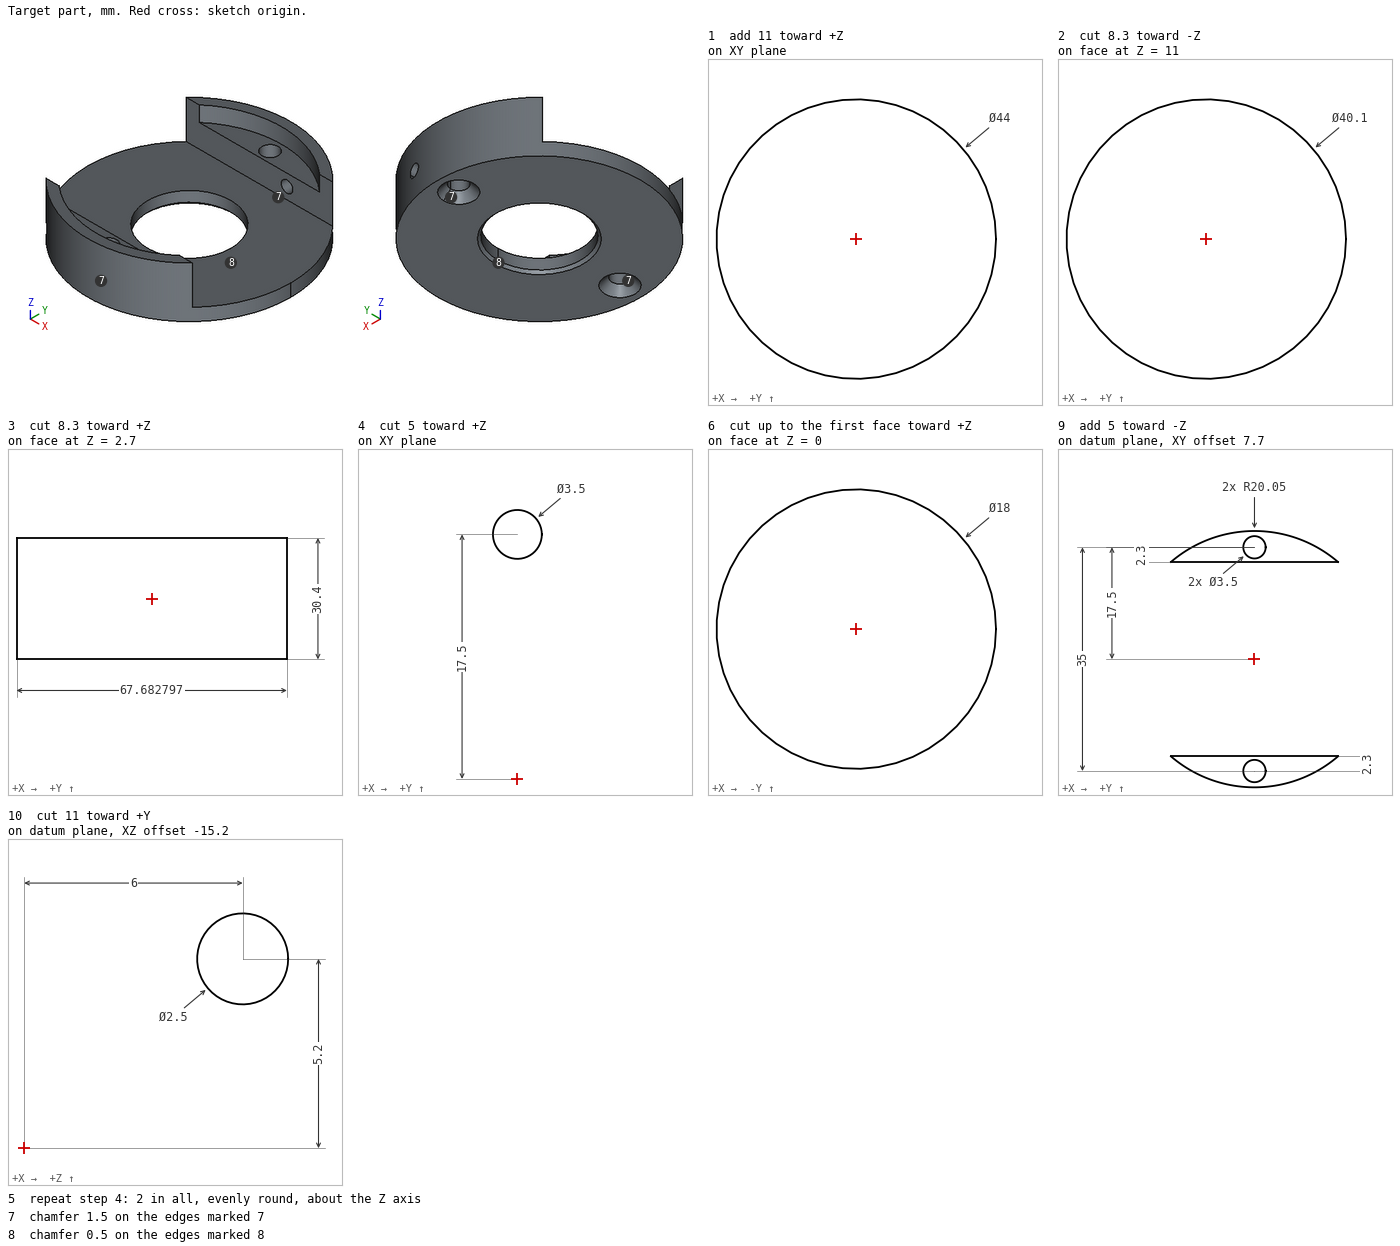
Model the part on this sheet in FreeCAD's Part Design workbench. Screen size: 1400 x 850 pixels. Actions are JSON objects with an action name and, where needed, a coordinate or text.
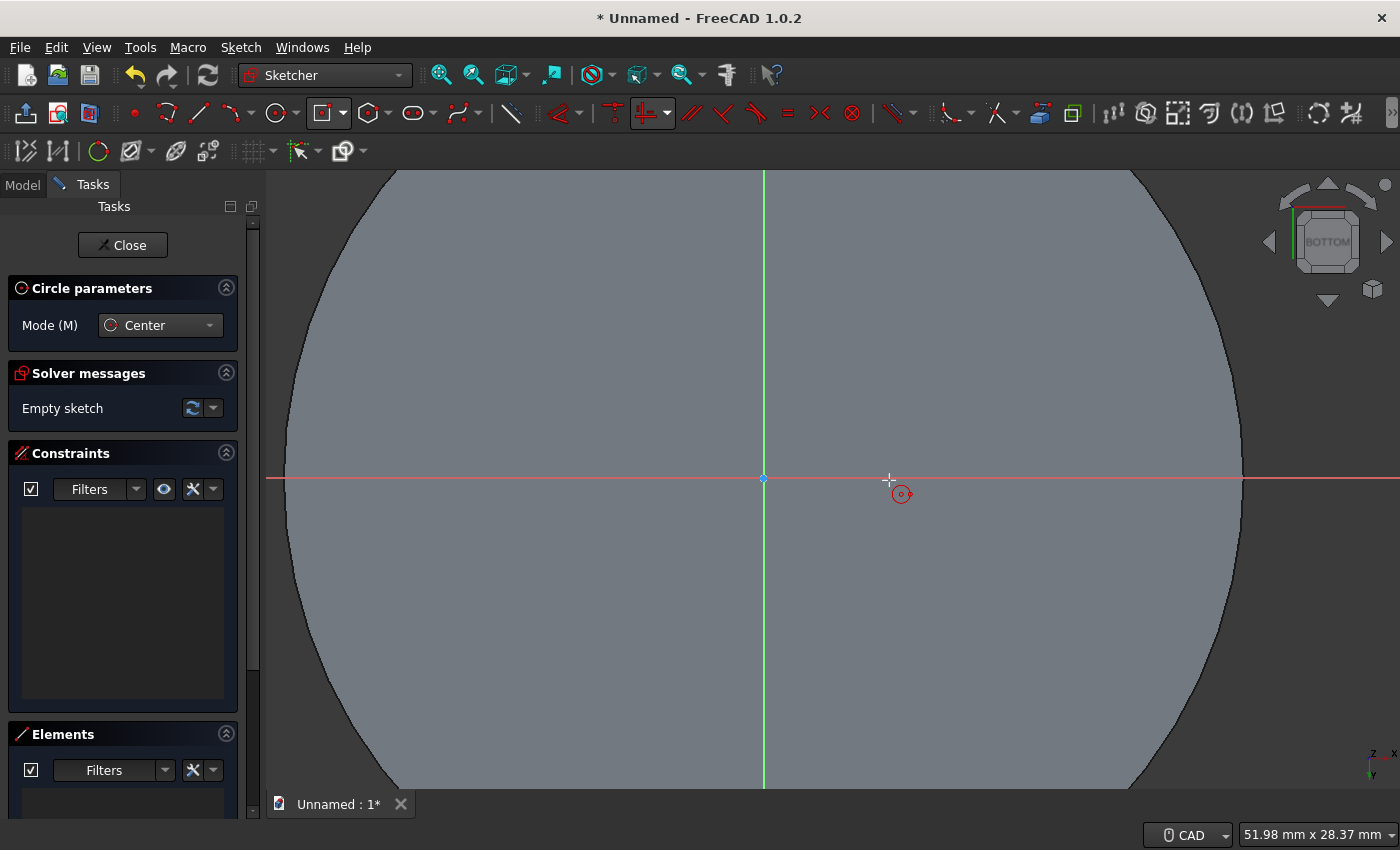
{"action": "left_click", "coordinate": [764, 478]}
{"action": "left_click", "coordinate": [903, 339]}
{"action": "key", "text": "Escape"}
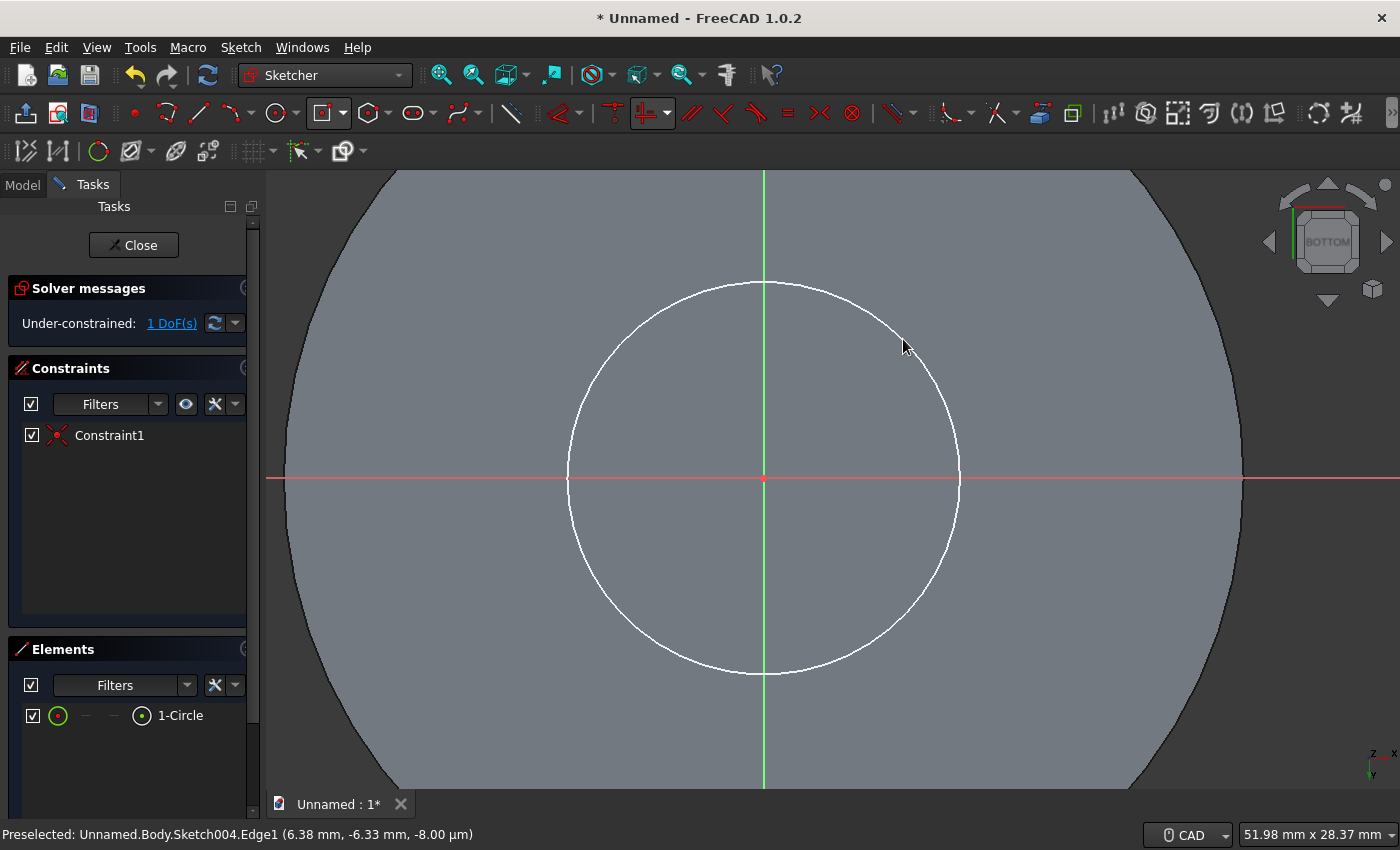
{"action": "key", "text": "d"}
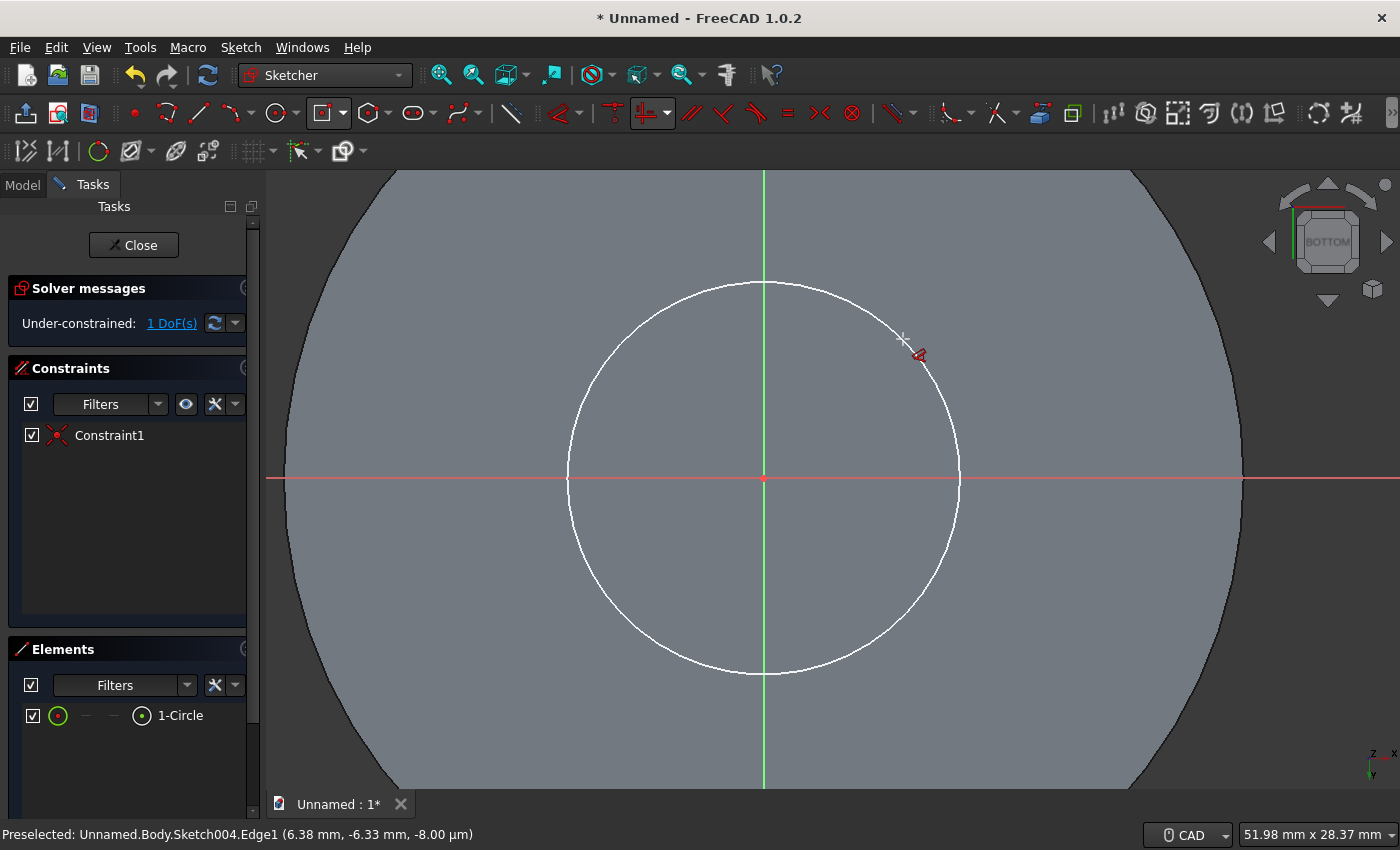
{"action": "left_click", "coordinate": [902, 339]}
{"action": "left_click", "coordinate": [925, 316]}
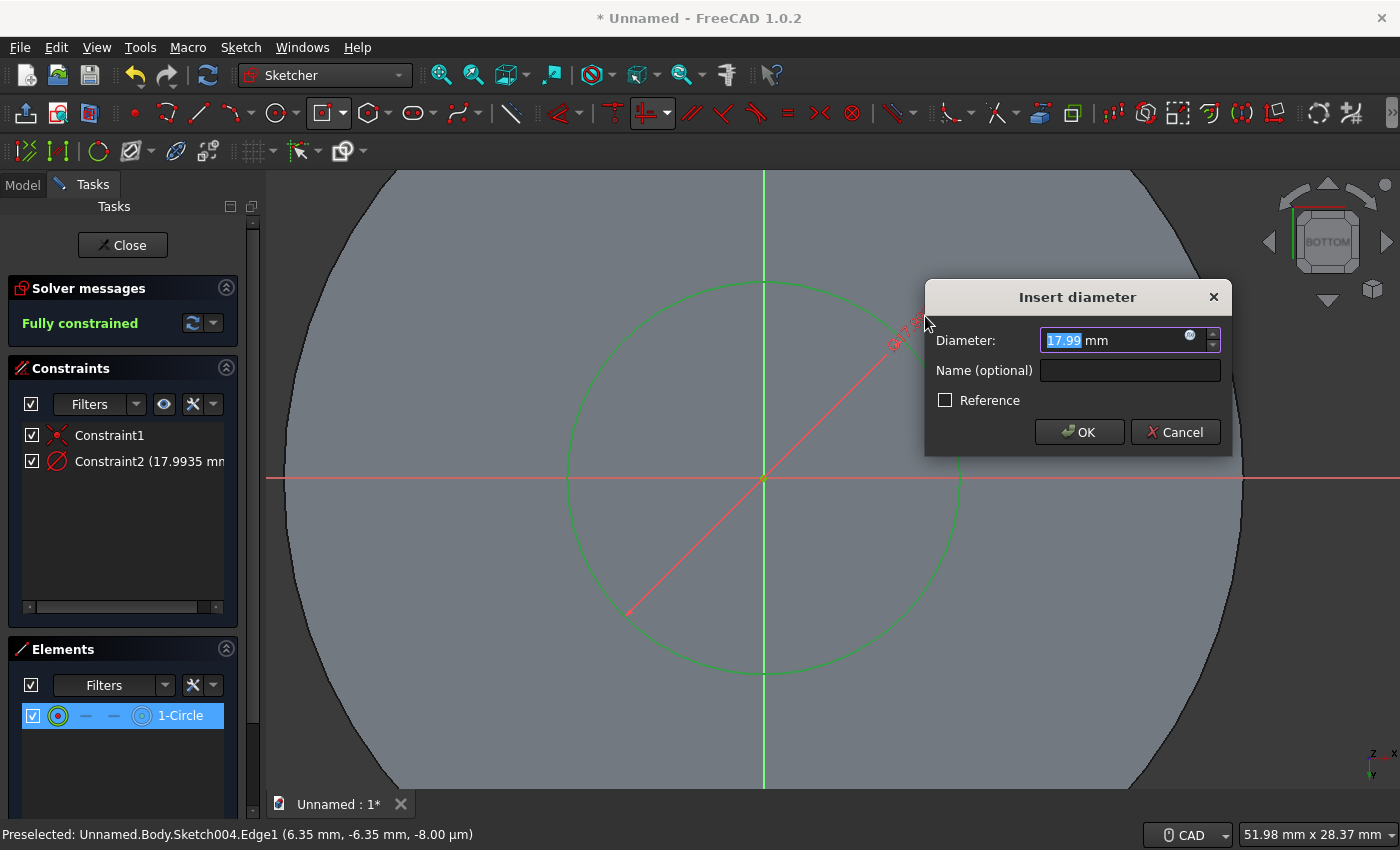
{"action": "type", "text": "18"}
{"action": "key", "text": "Return"}
{"action": "key", "text": "Escape"}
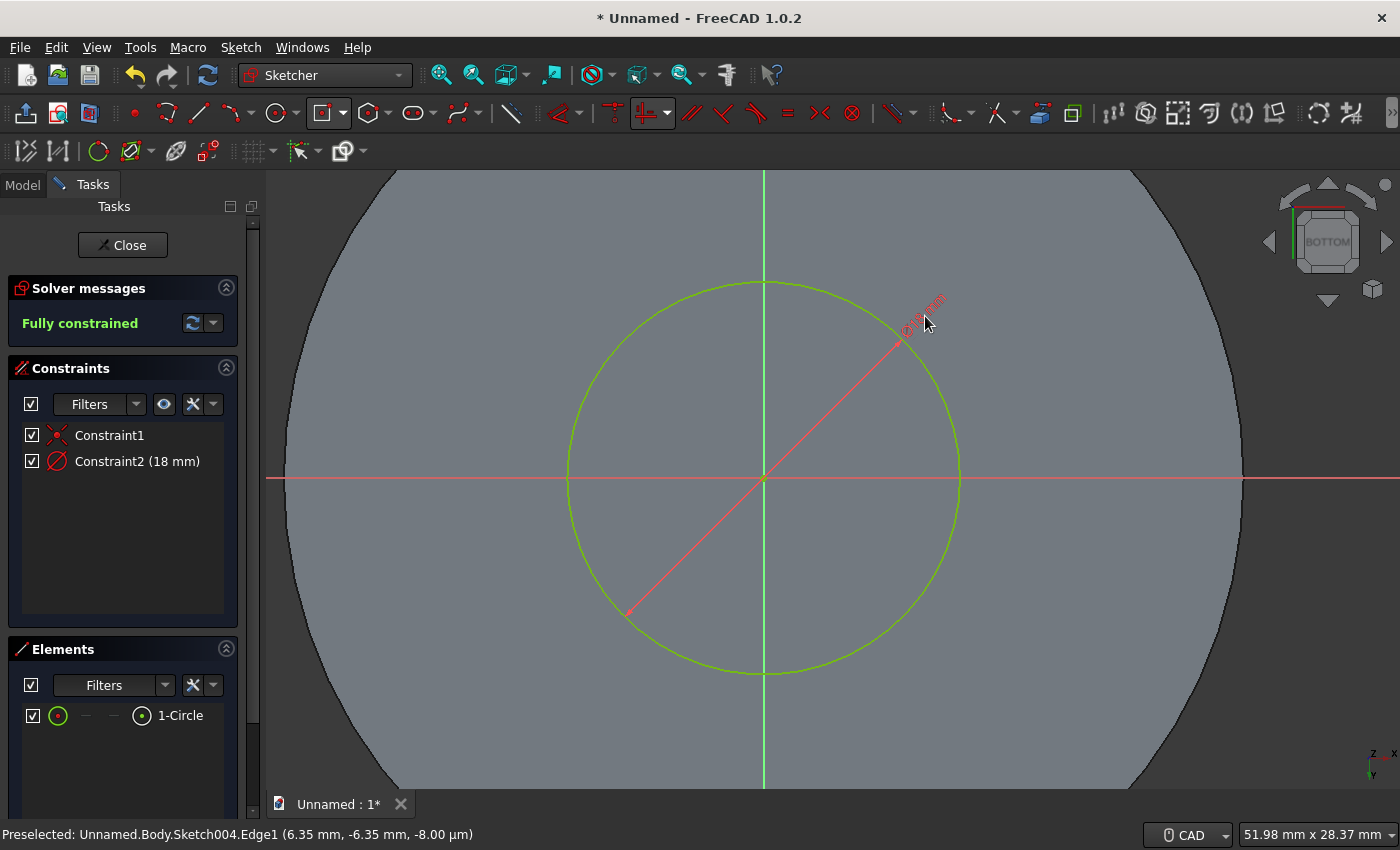
{"action": "left_click", "coordinate": [123, 245]}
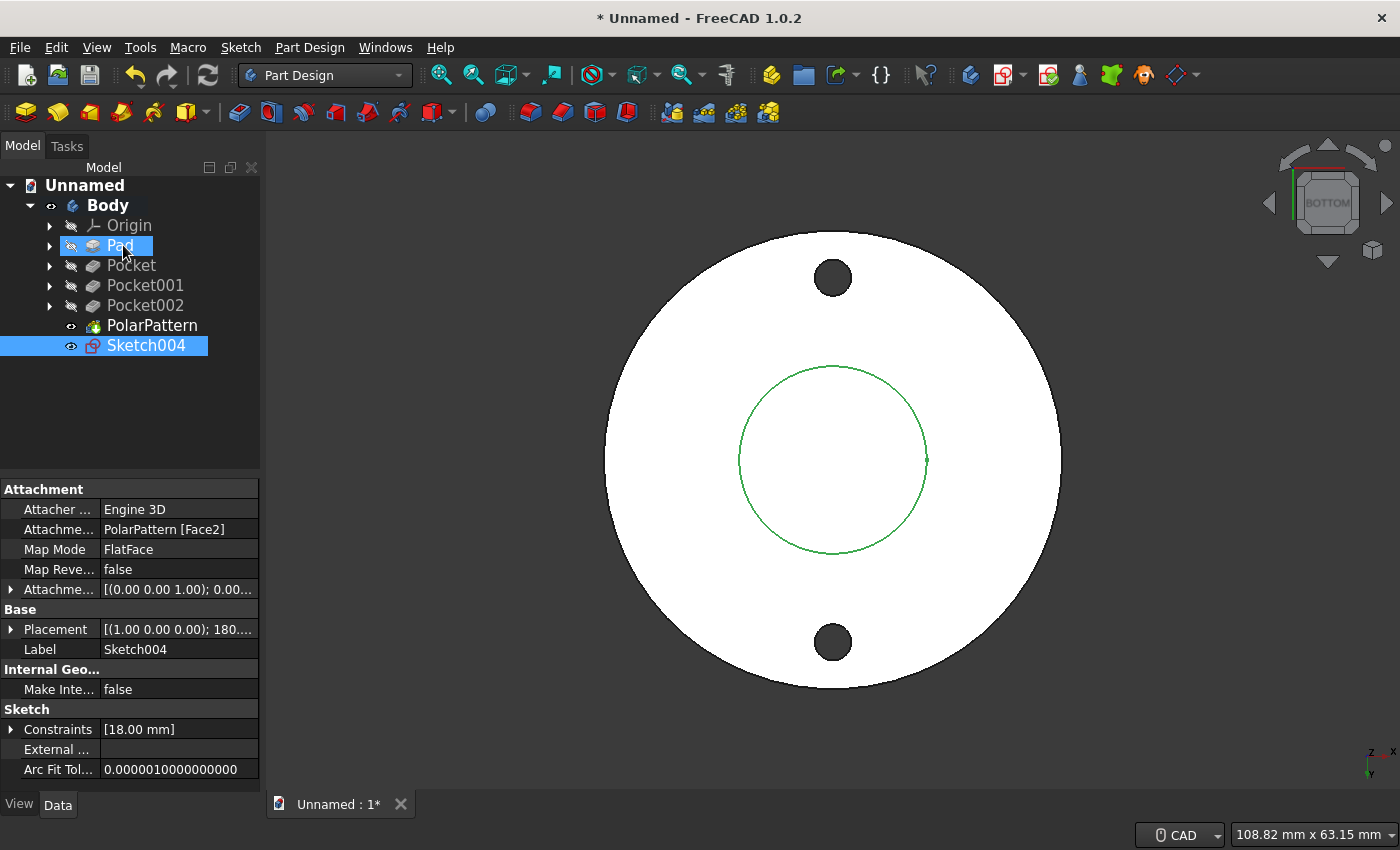
{"action": "left_click", "coordinate": [240, 112]}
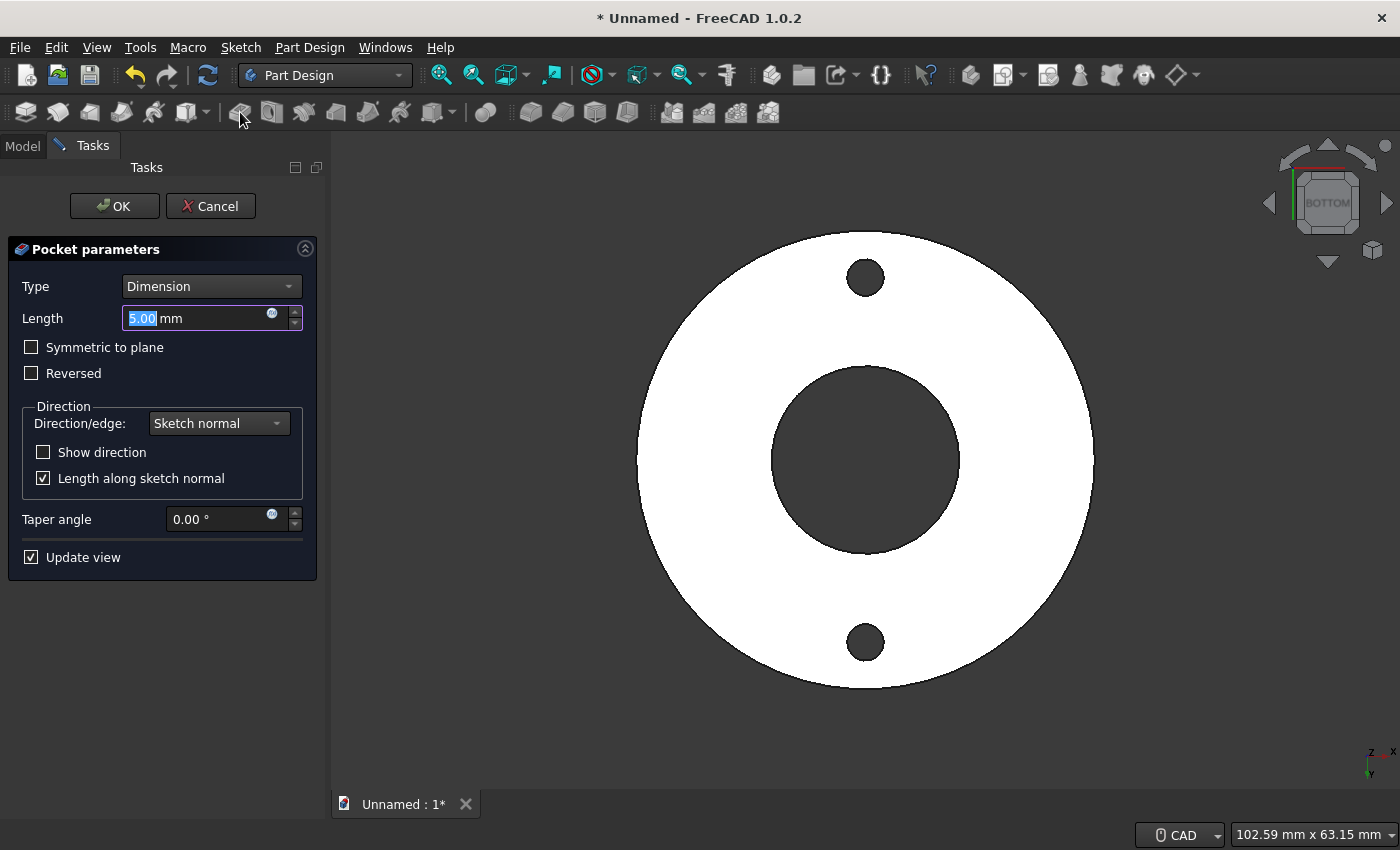
{"action": "left_click", "coordinate": [212, 286]}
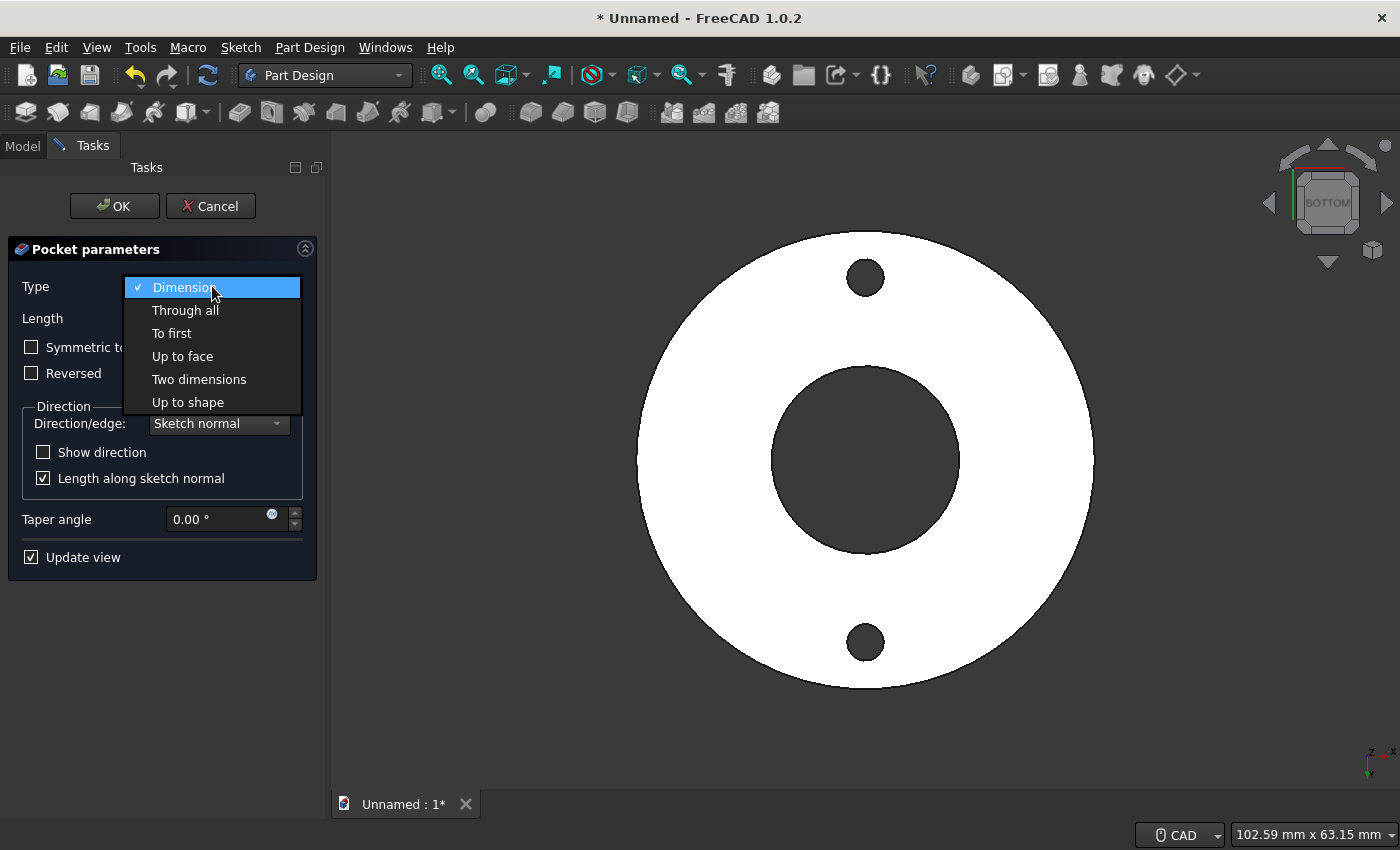
{"action": "left_click", "coordinate": [212, 334]}